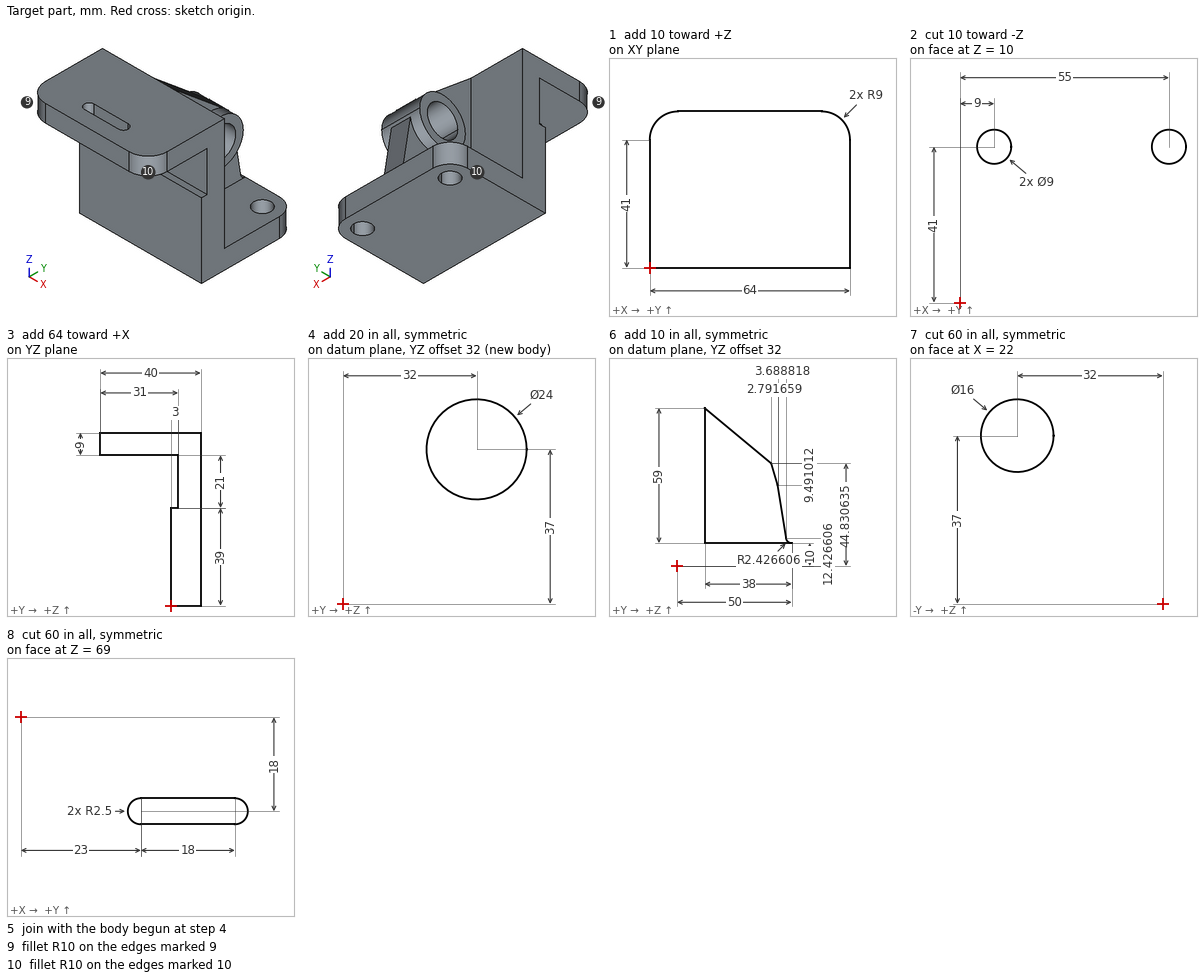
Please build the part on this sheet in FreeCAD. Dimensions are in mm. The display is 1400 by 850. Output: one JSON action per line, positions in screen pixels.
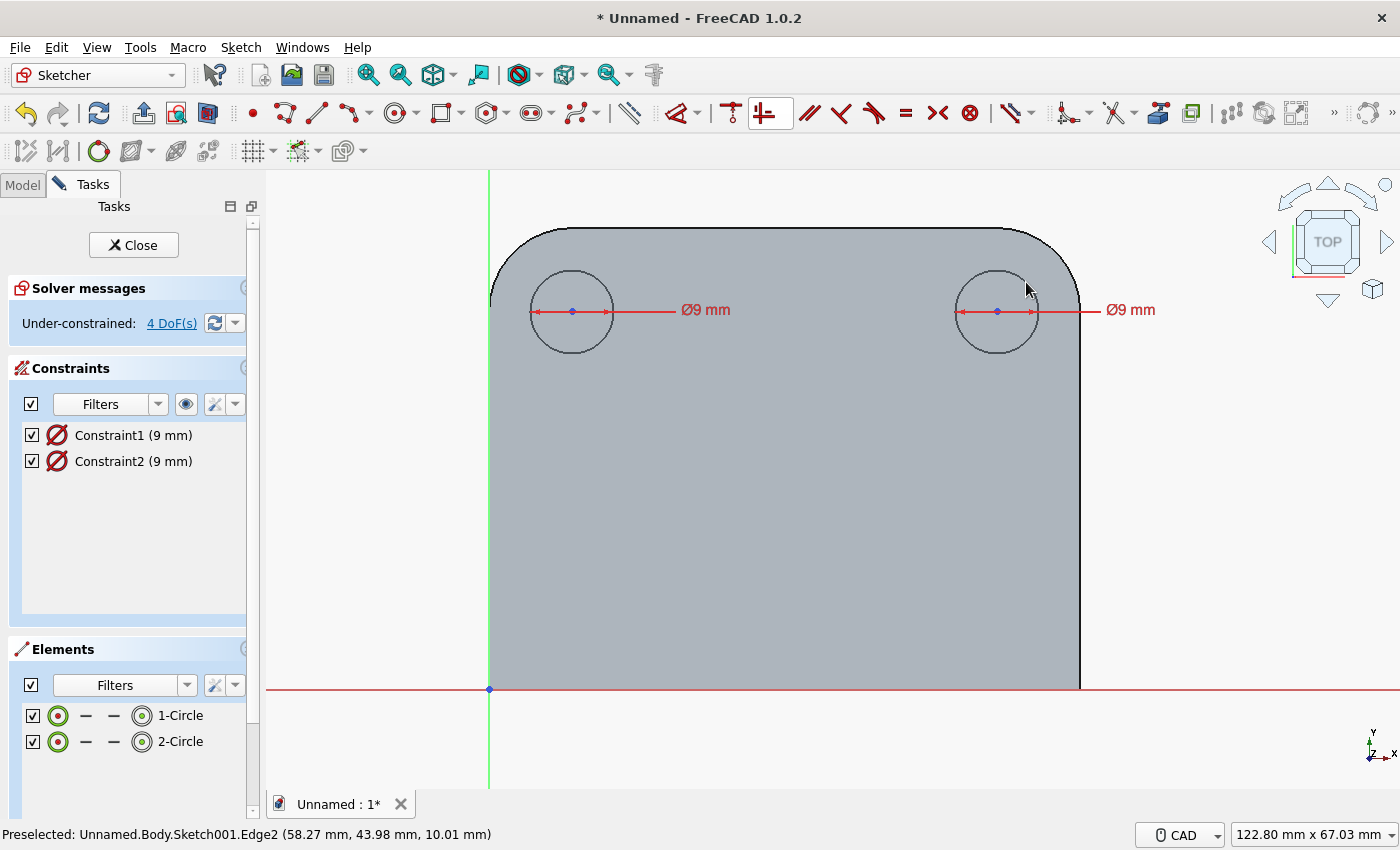
{"action": "left_click", "coordinate": [572, 312]}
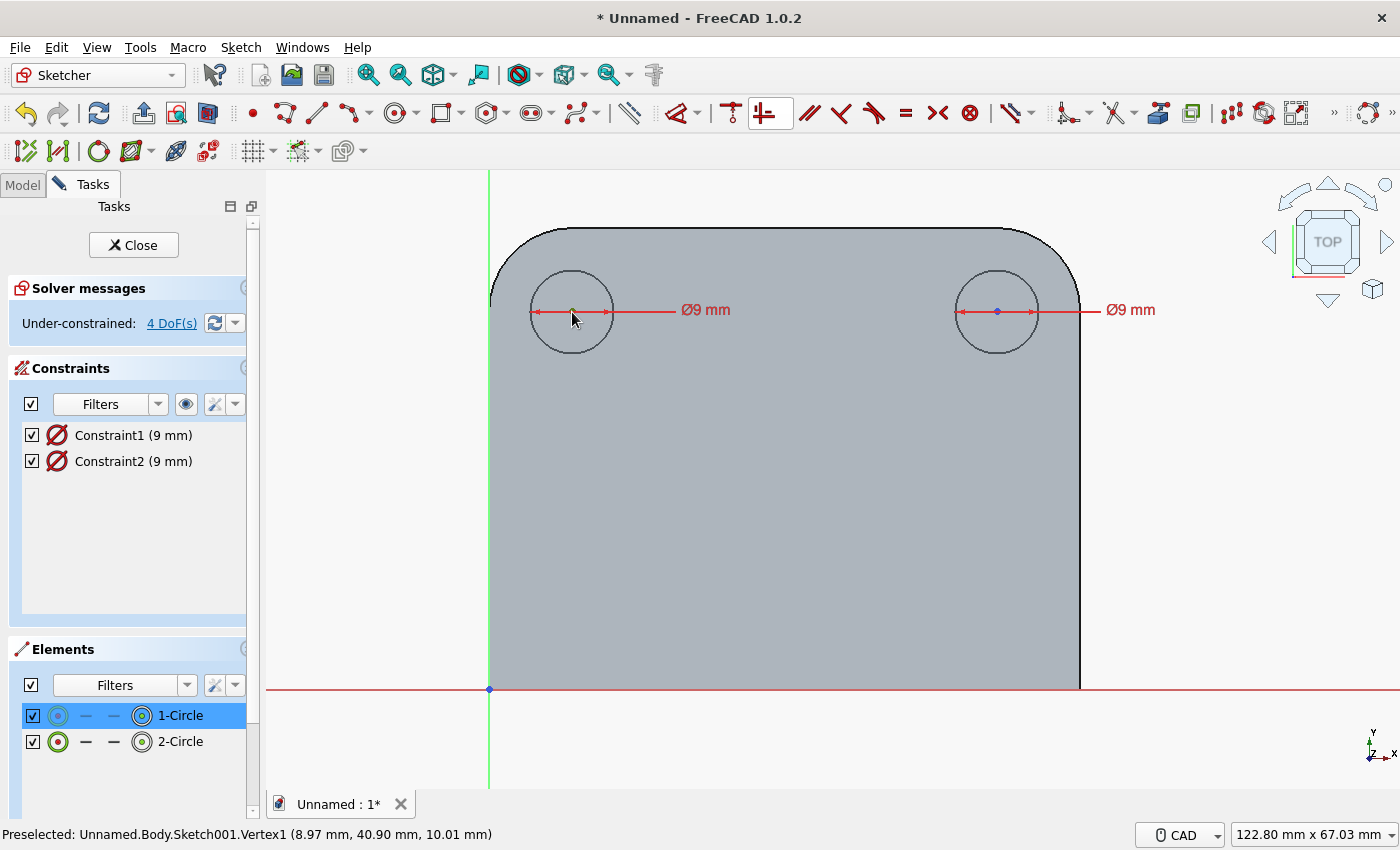
{"action": "left_click", "coordinate": [997, 312]}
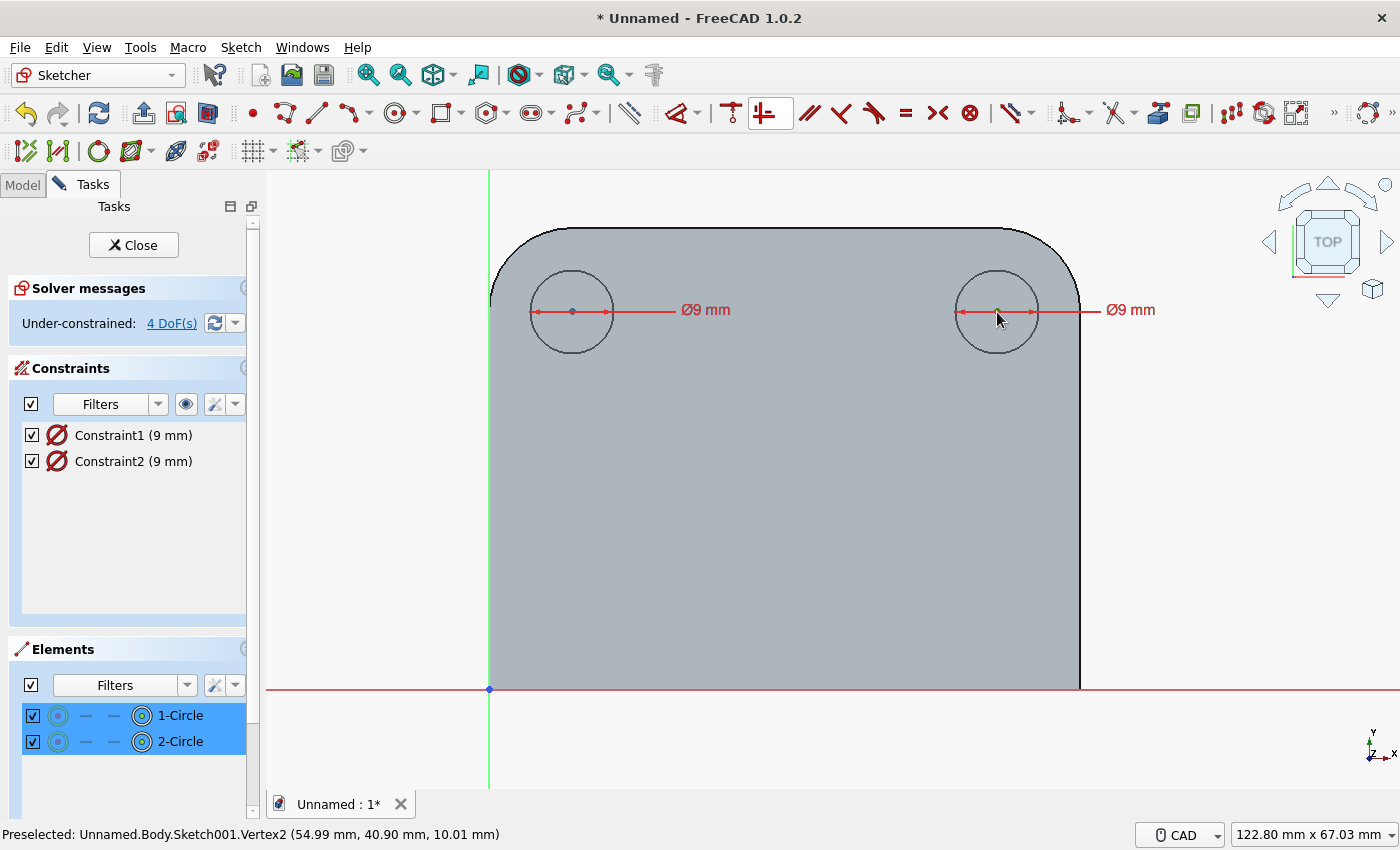
{"action": "left_click", "coordinate": [788, 114]}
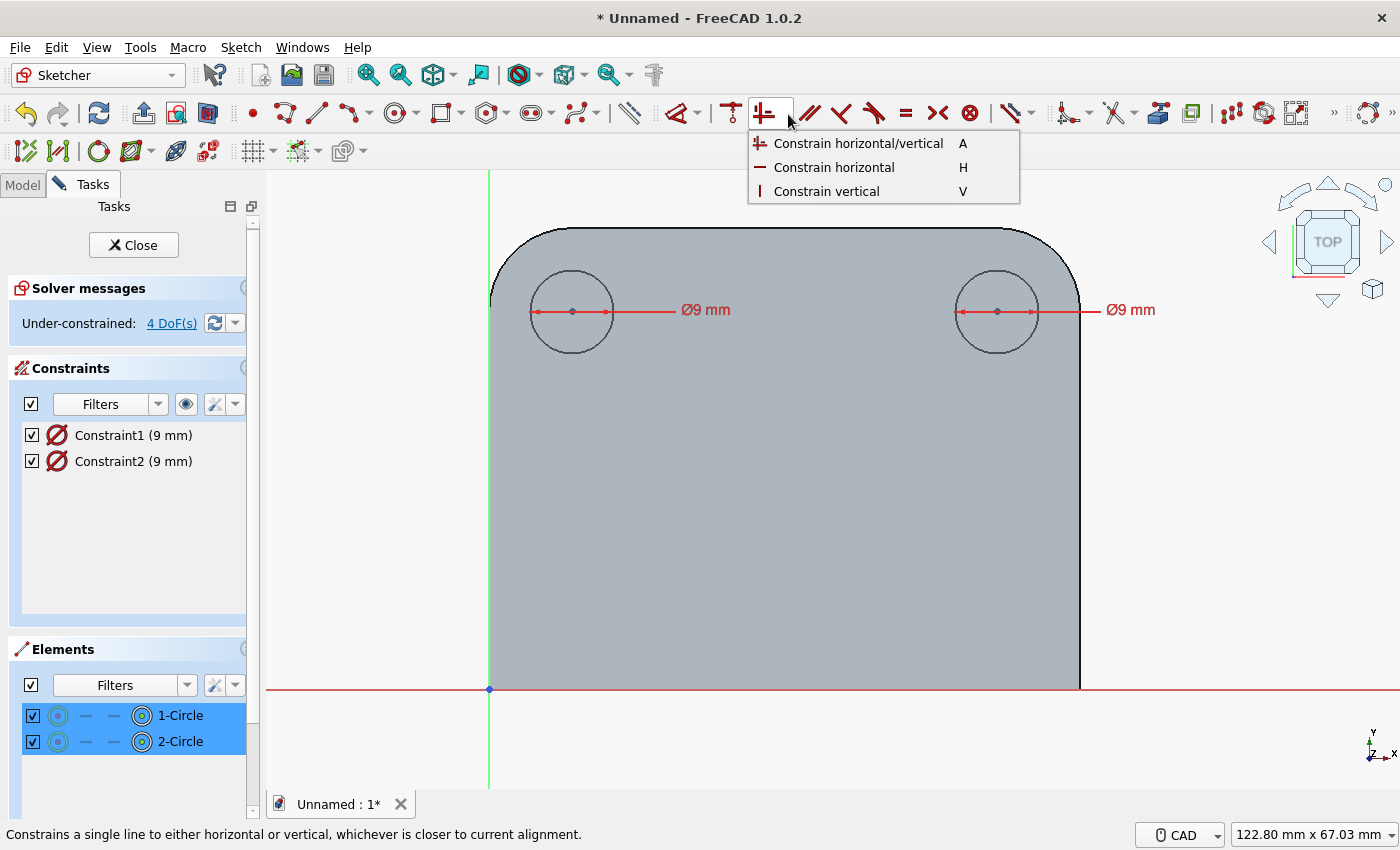
{"action": "left_click", "coordinate": [884, 167]}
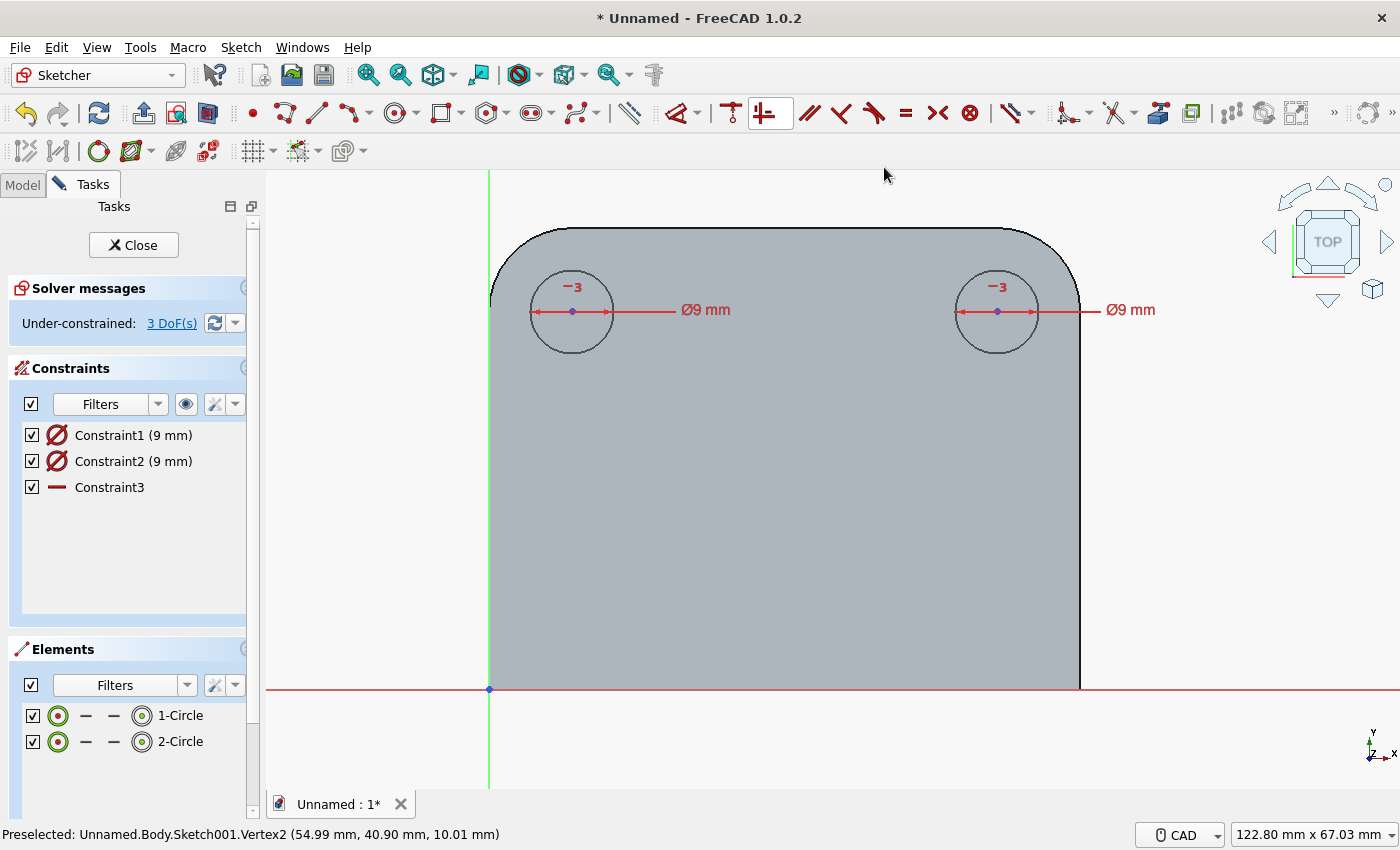
{"action": "left_click", "coordinate": [676, 114]}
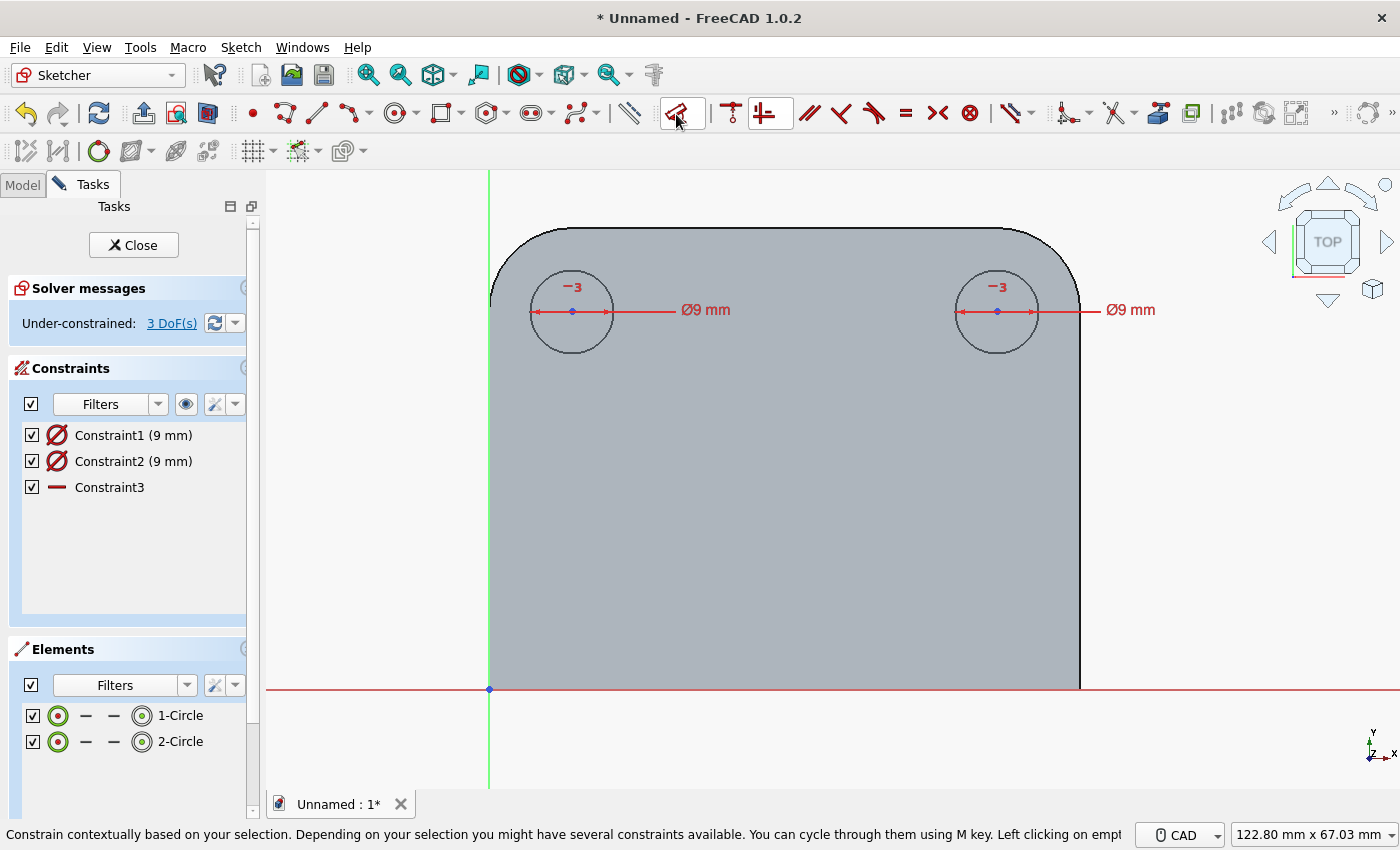
{"action": "left_click", "coordinate": [572, 312]}
{"action": "left_click", "coordinate": [531, 724]}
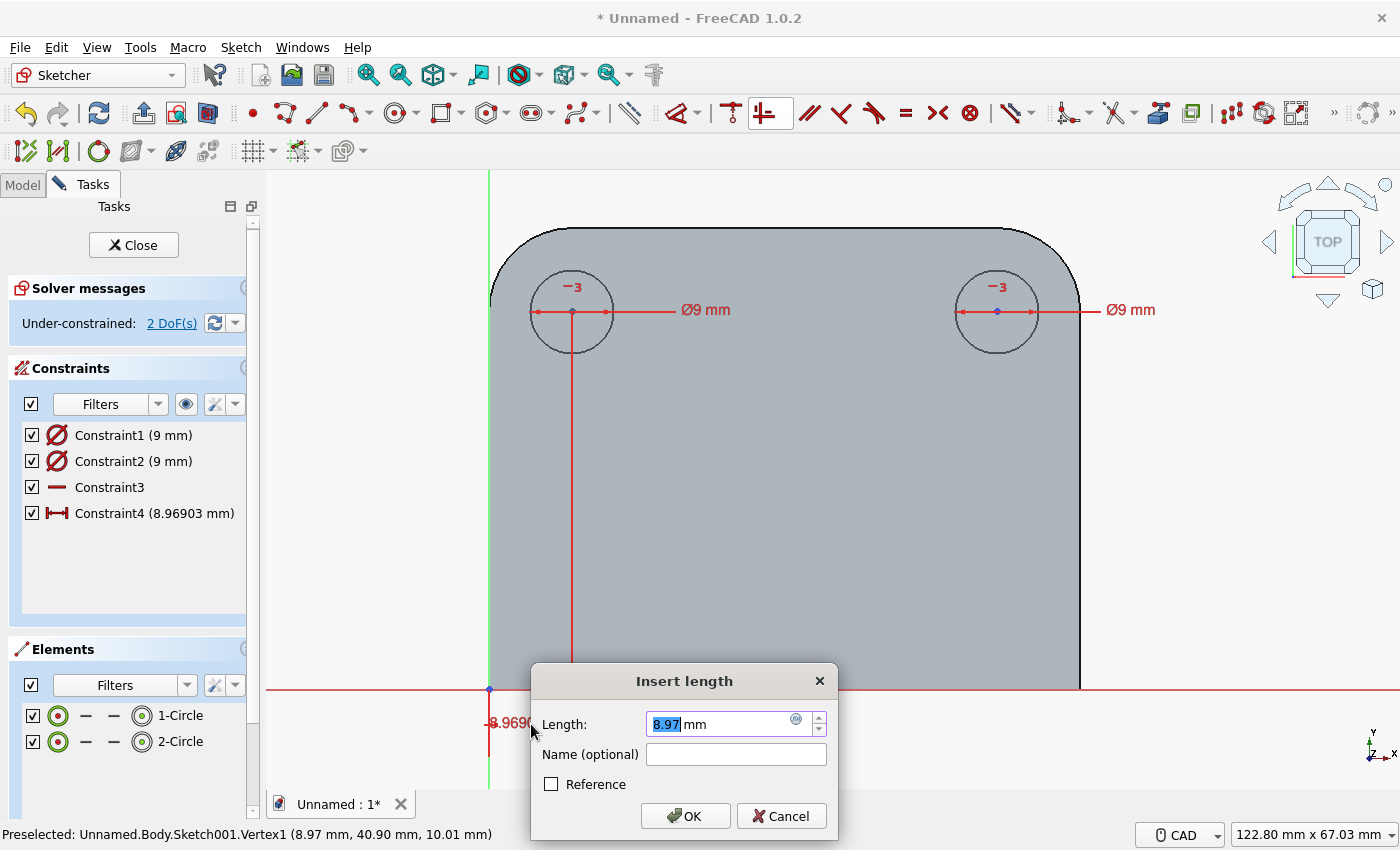
{"action": "type", "text": "9"}
{"action": "key", "text": "Return"}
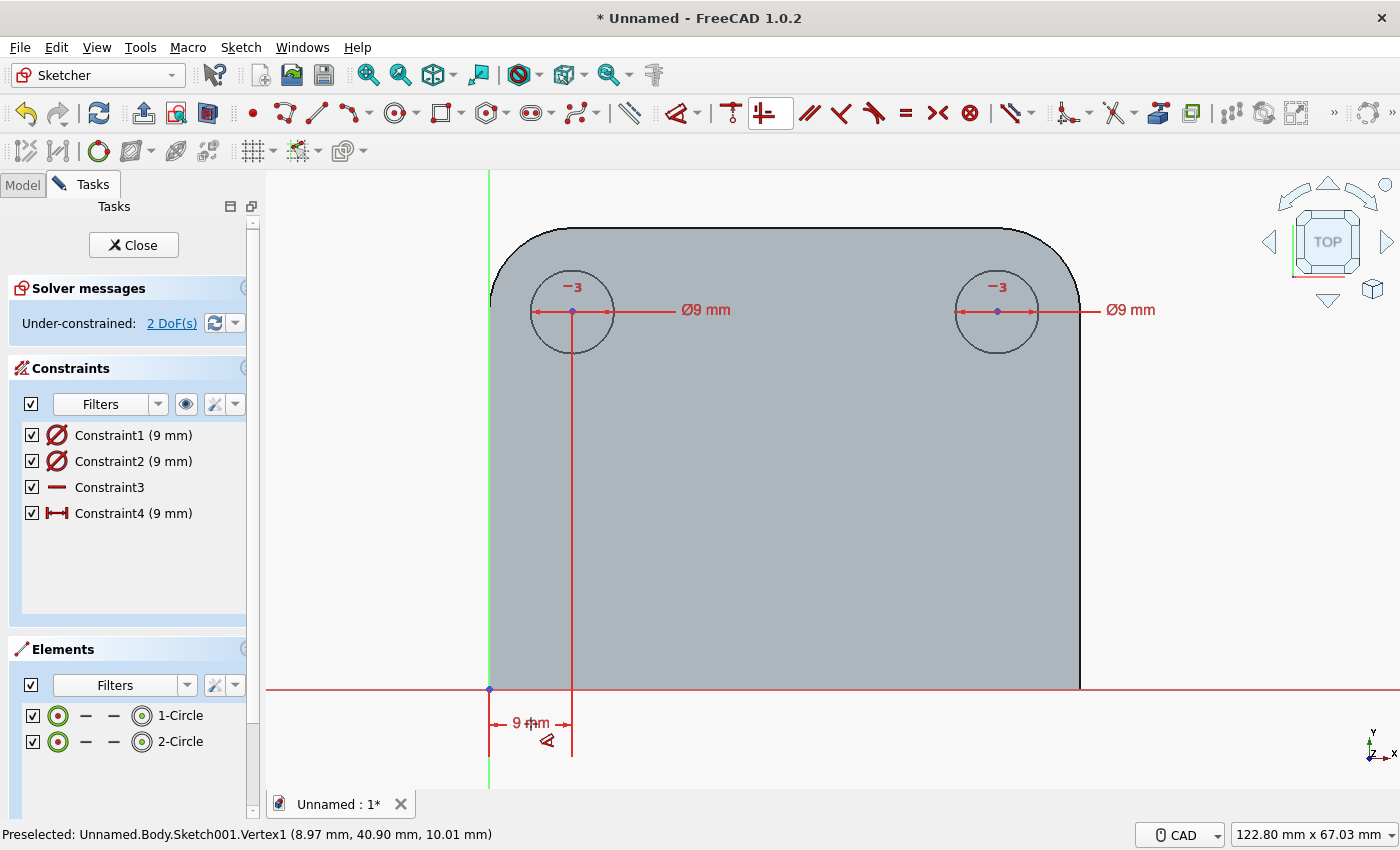
{"action": "left_click", "coordinate": [572, 312]}
{"action": "left_click", "coordinate": [455, 501]}